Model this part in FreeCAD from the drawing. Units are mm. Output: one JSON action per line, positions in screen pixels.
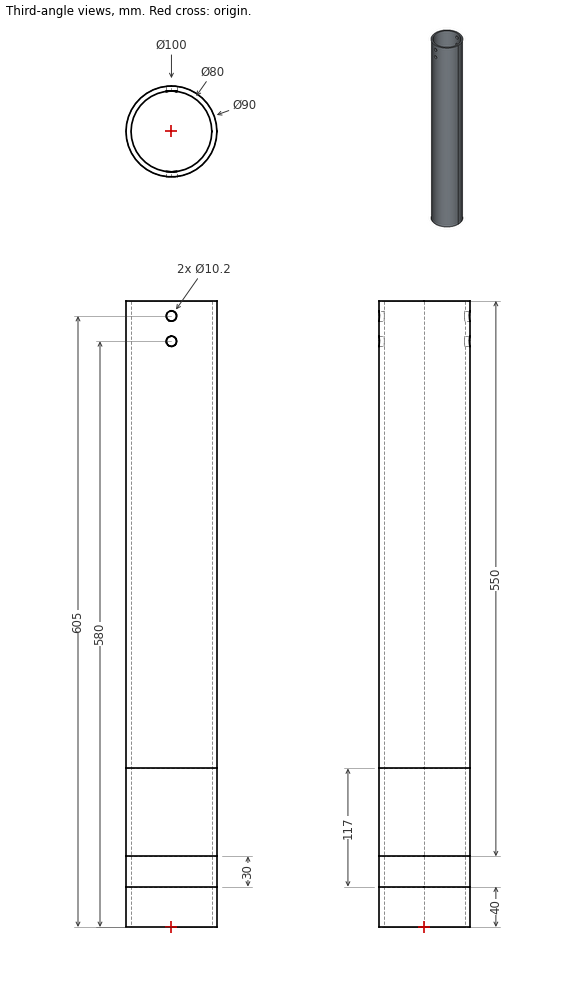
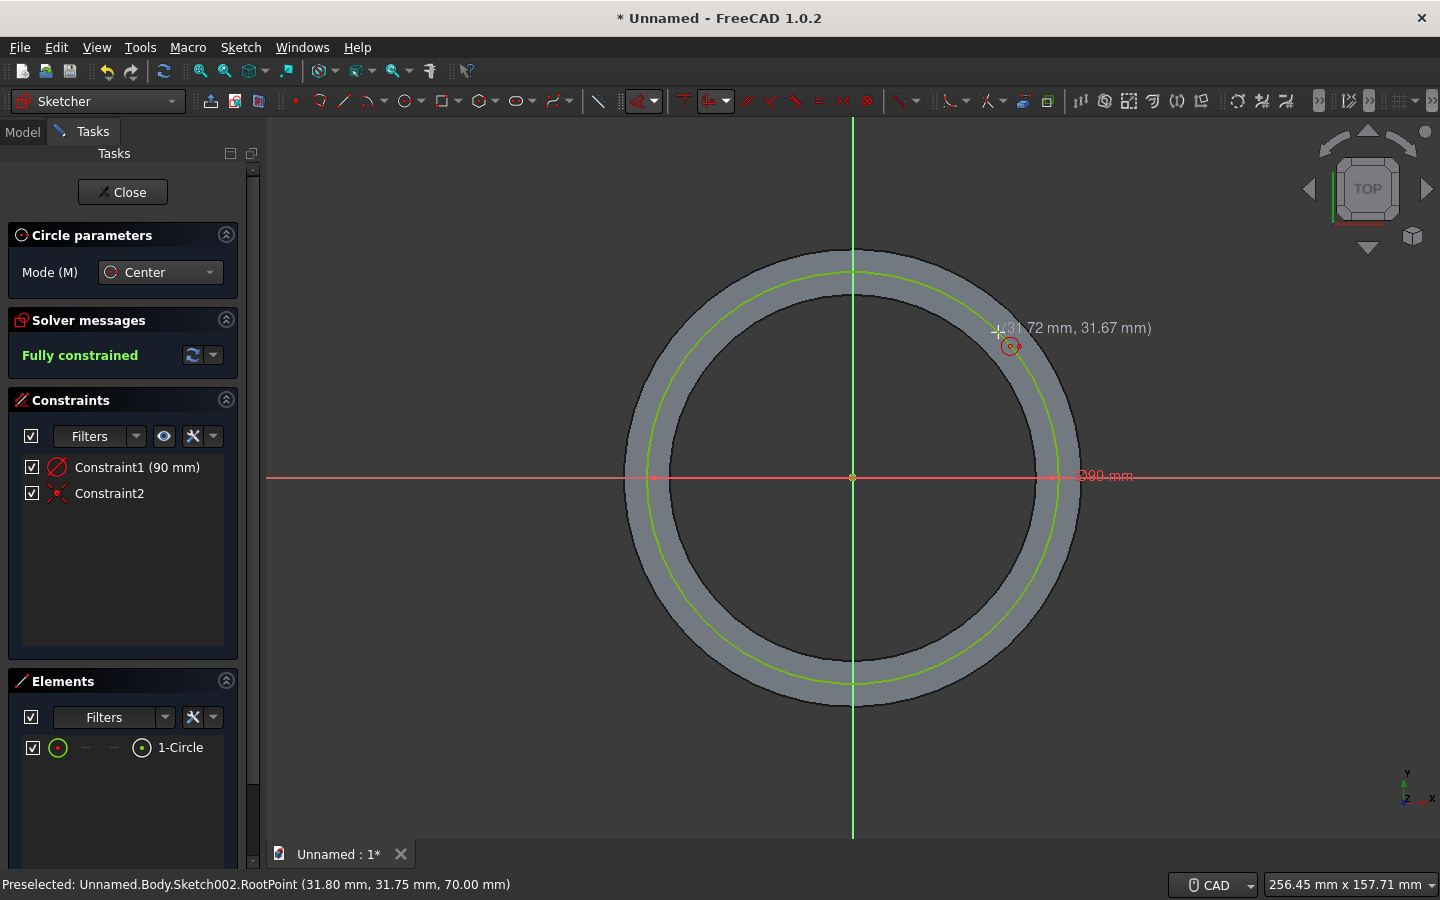
{"action": "left_click", "coordinate": [853, 478]}
{"action": "mouse_move", "coordinate": [982, 349]}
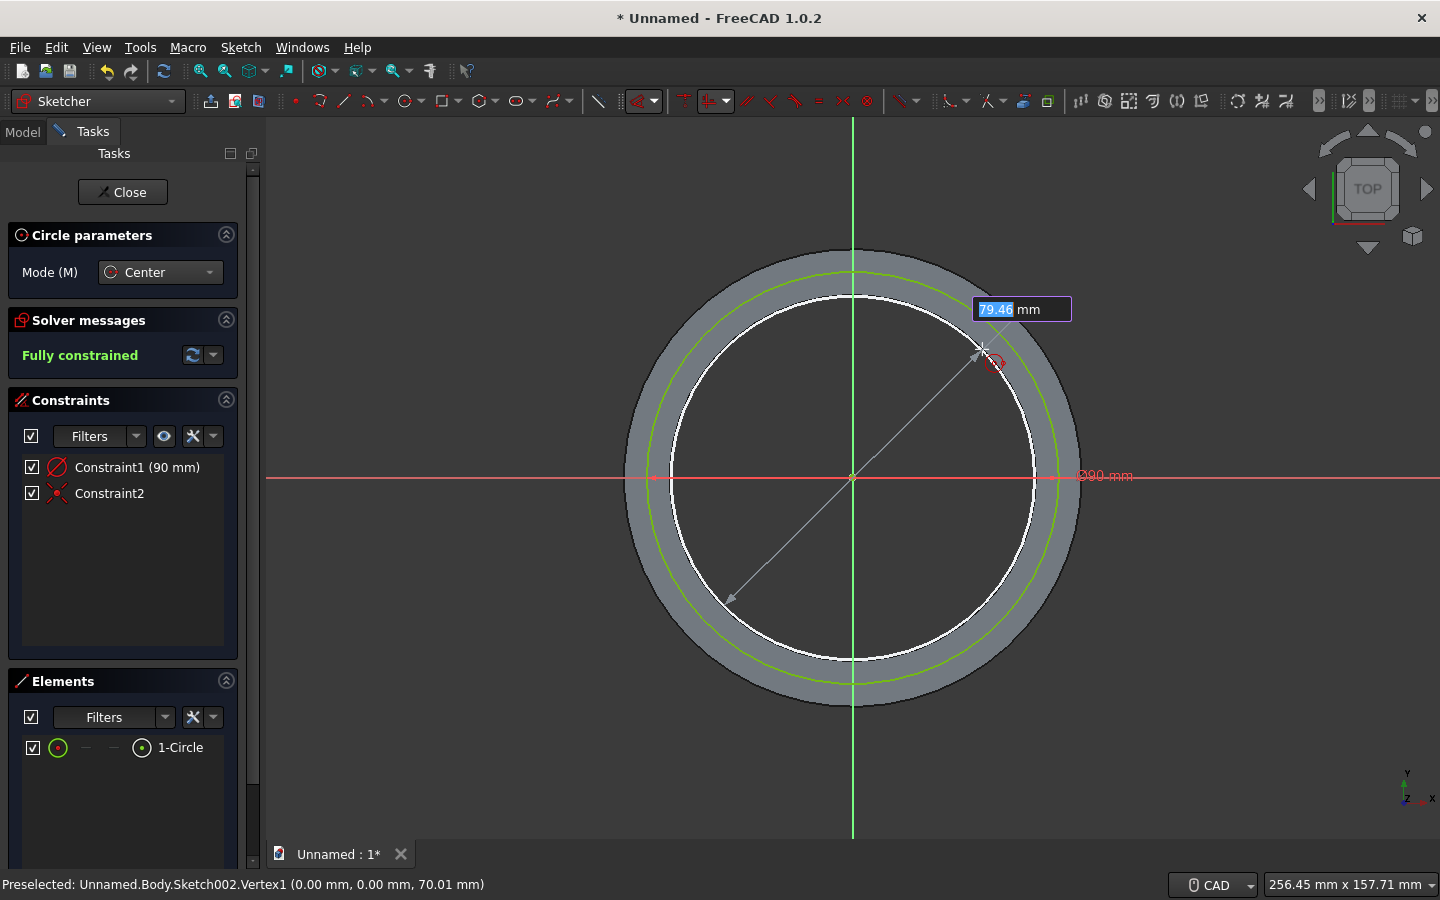
{"action": "type", "text": "80"}
{"action": "key", "text": "Return"}
{"action": "key", "text": "Escape"}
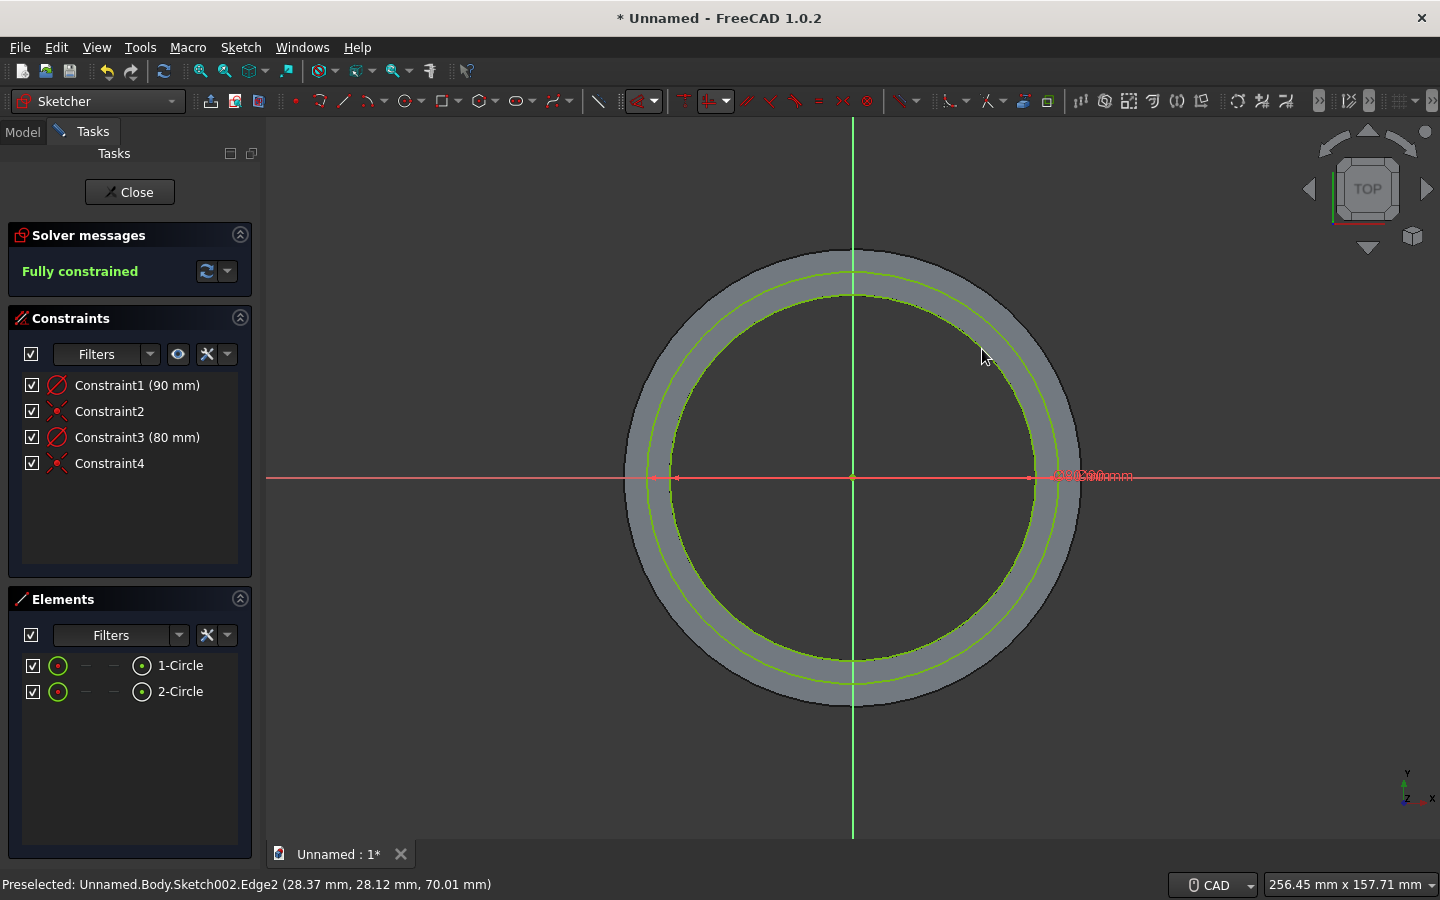
{"action": "left_click", "coordinate": [130, 192]}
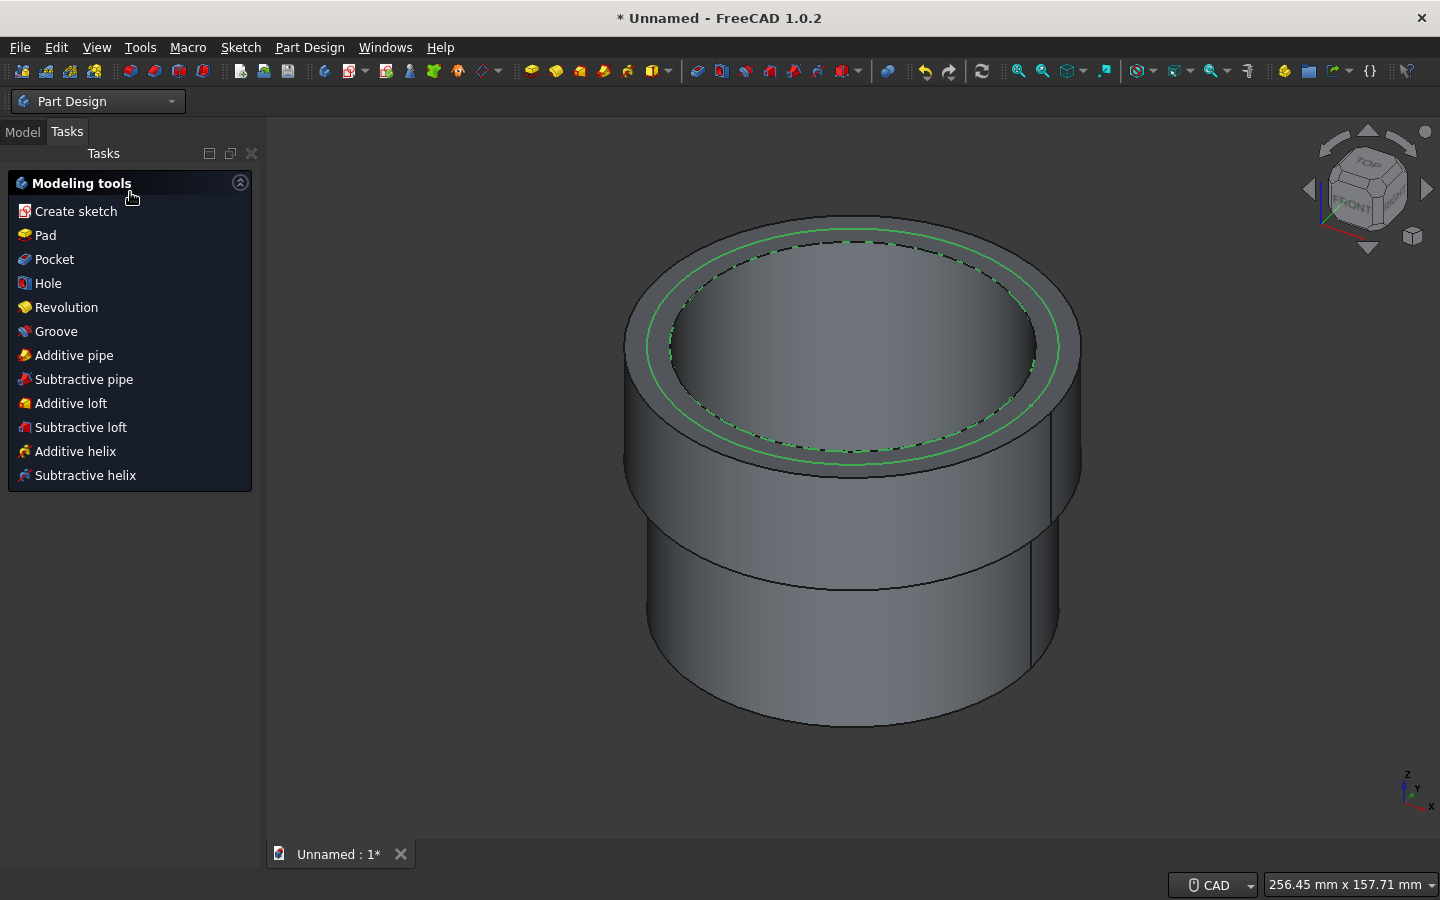
{"action": "left_click", "coordinate": [532, 72]}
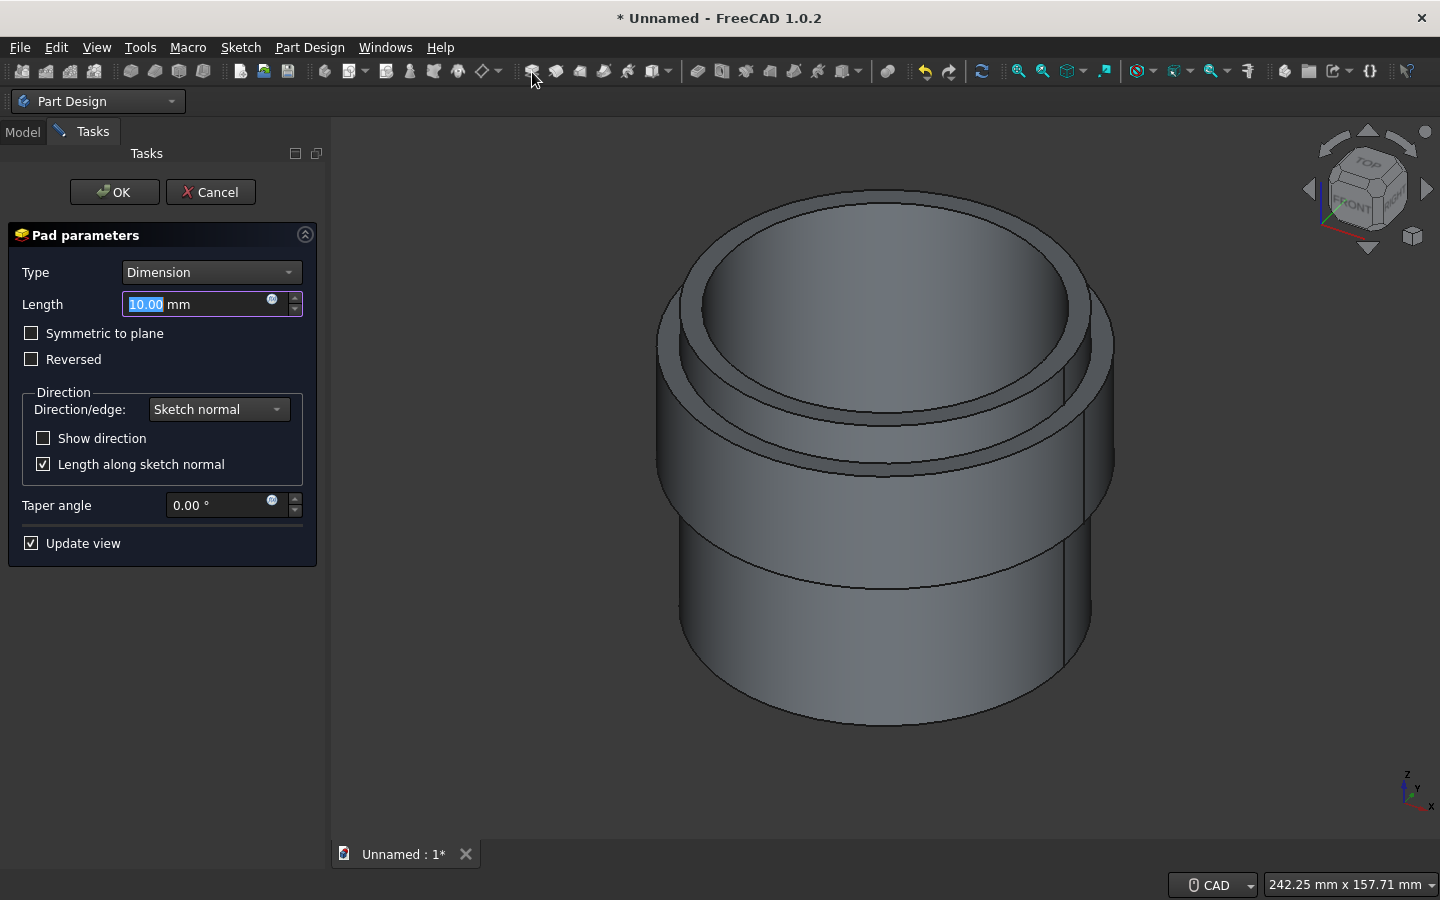
{"action": "type", "text": "550"}
{"action": "key", "text": "Tab"}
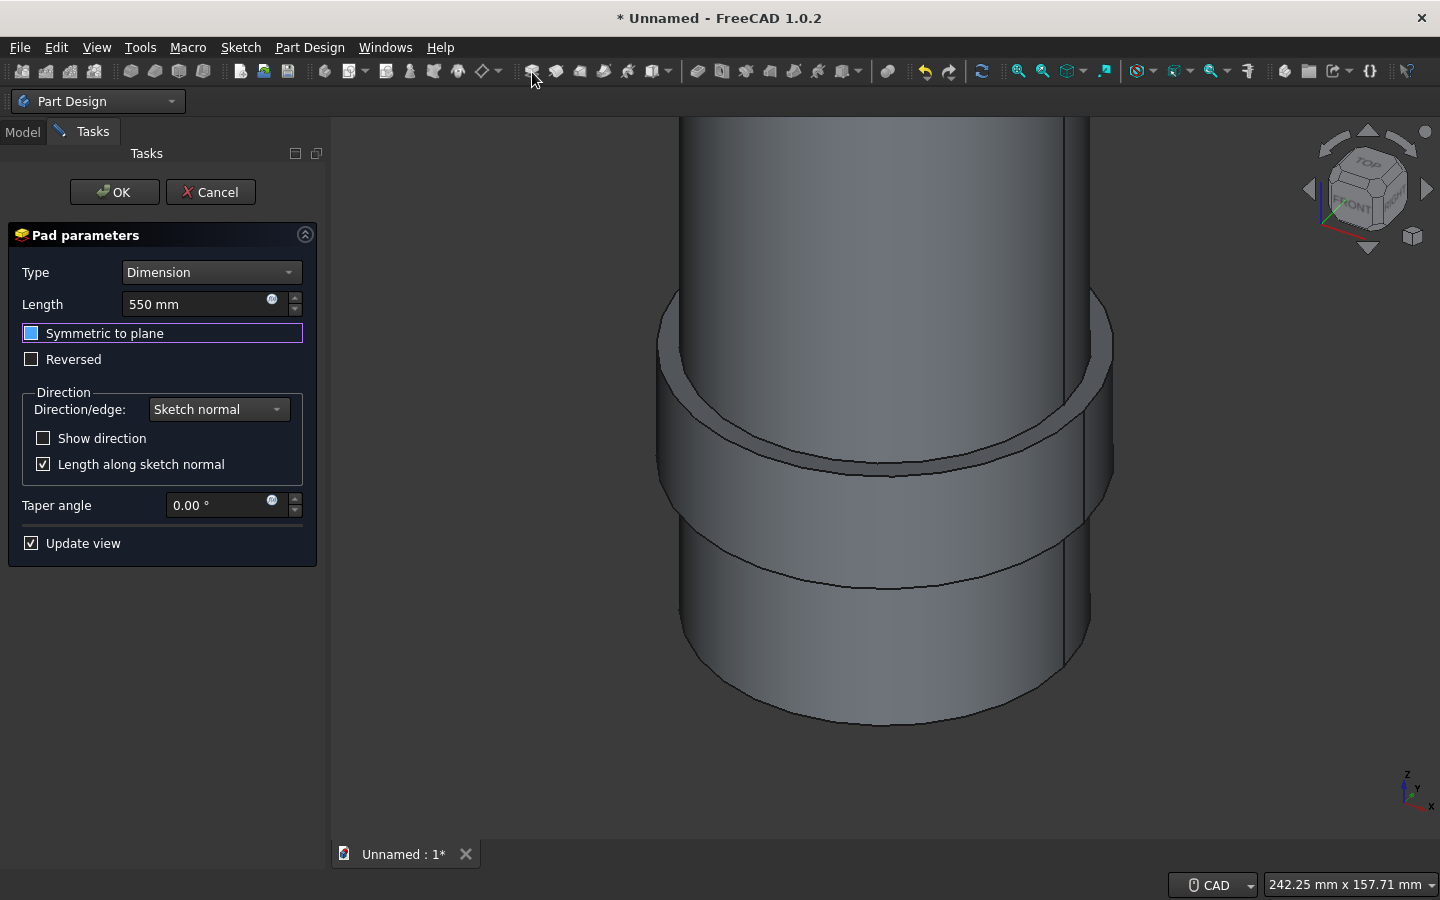
{"action": "left_click", "coordinate": [115, 192]}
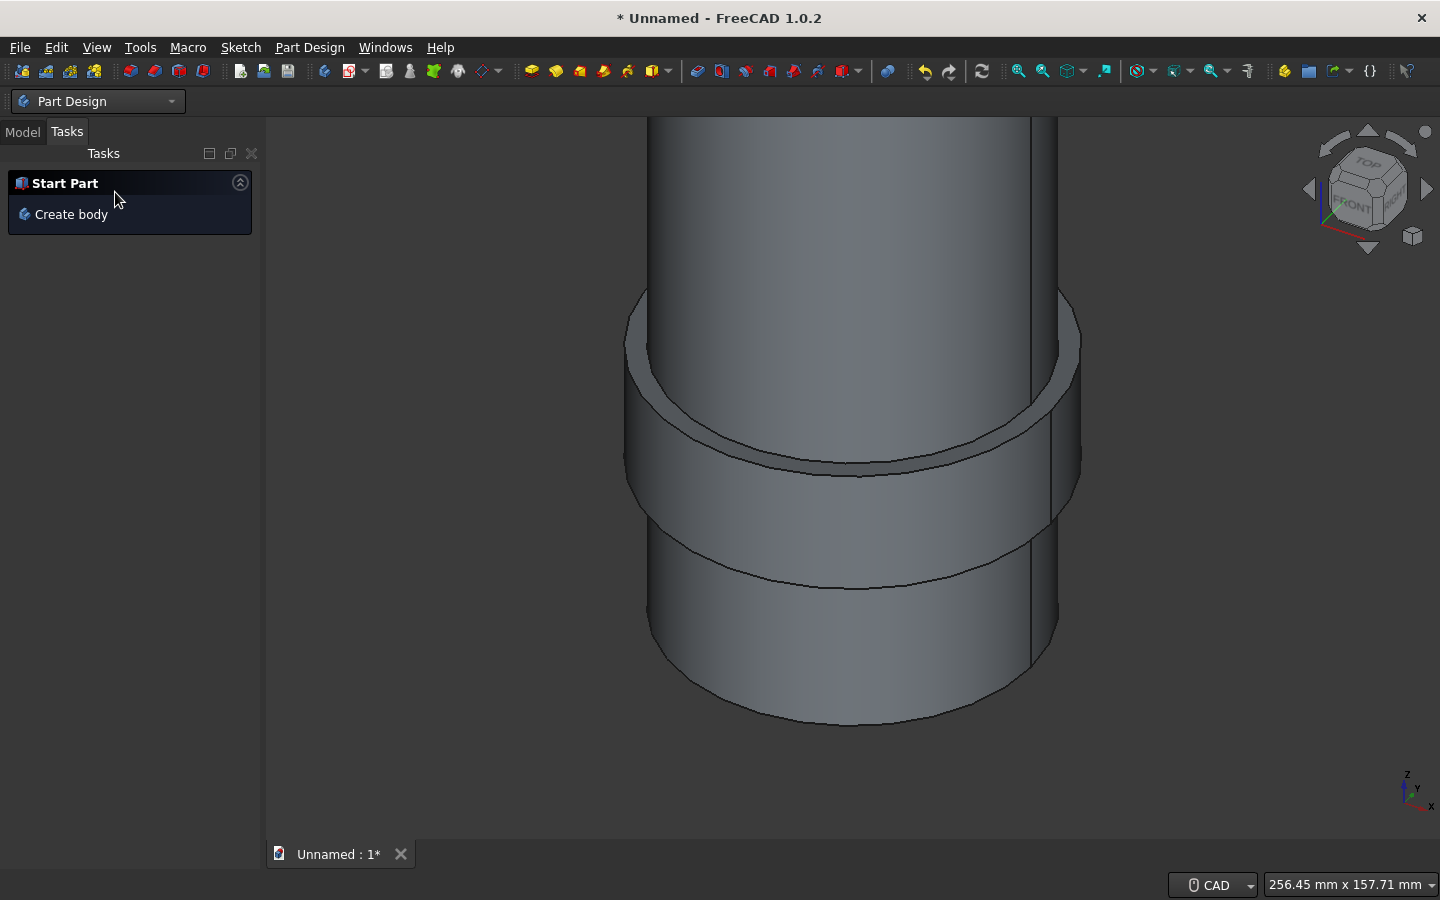
{"action": "left_click", "coordinate": [1020, 72]}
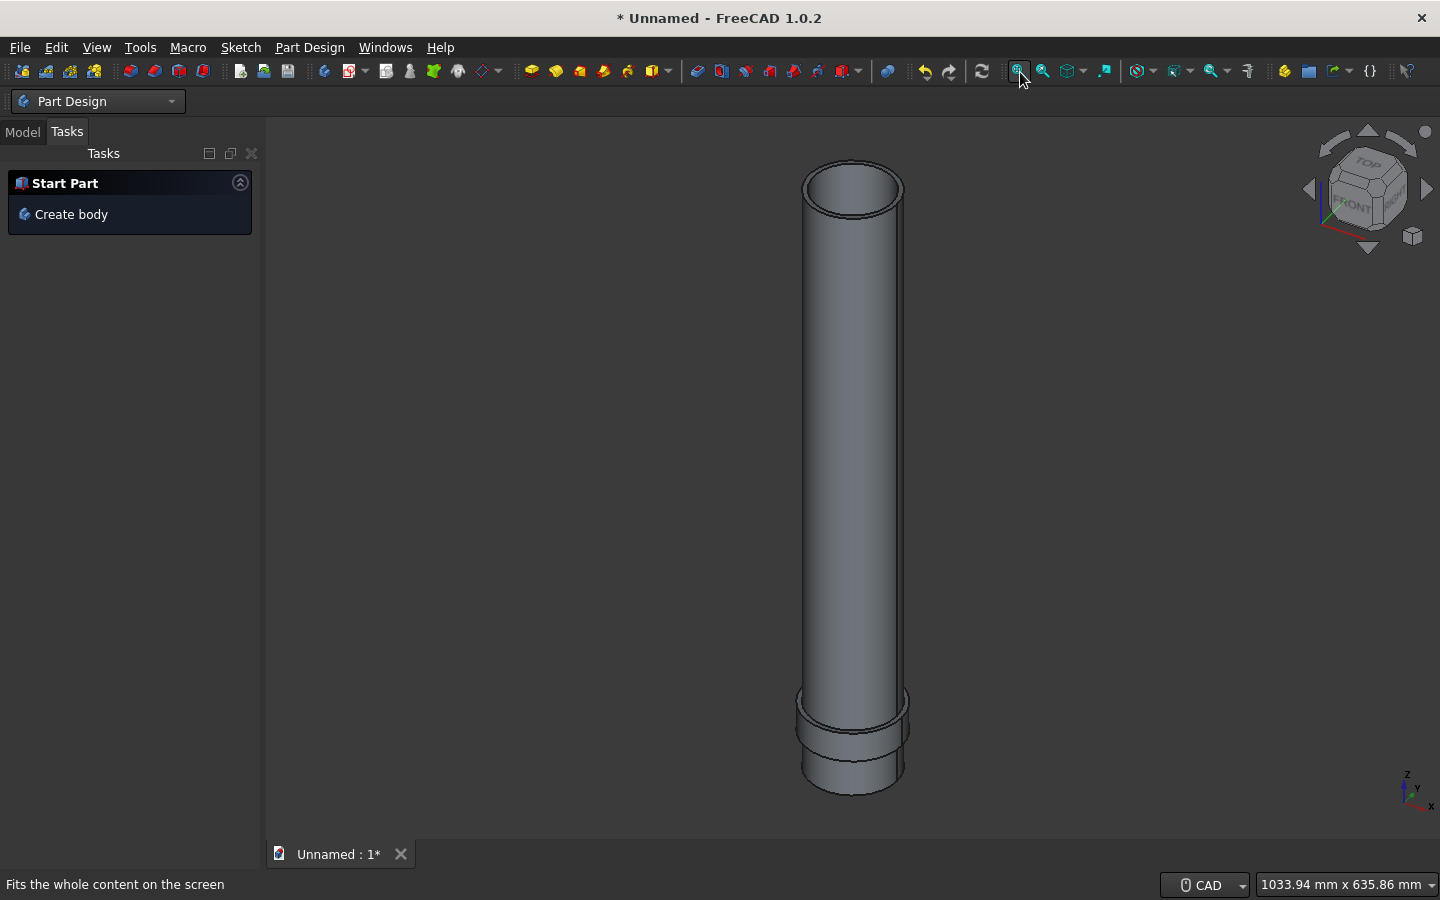
{"action": "left_click", "coordinate": [350, 72]}